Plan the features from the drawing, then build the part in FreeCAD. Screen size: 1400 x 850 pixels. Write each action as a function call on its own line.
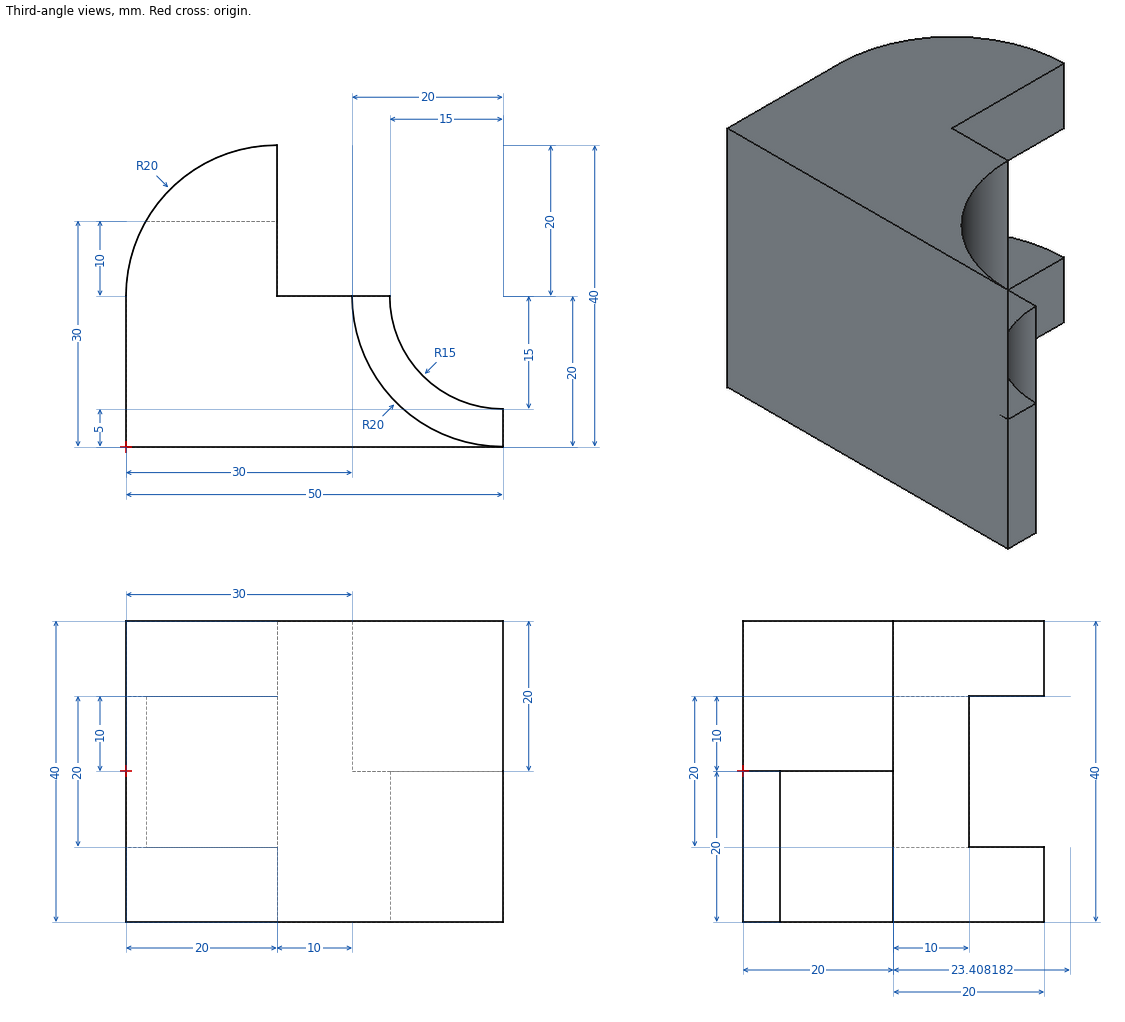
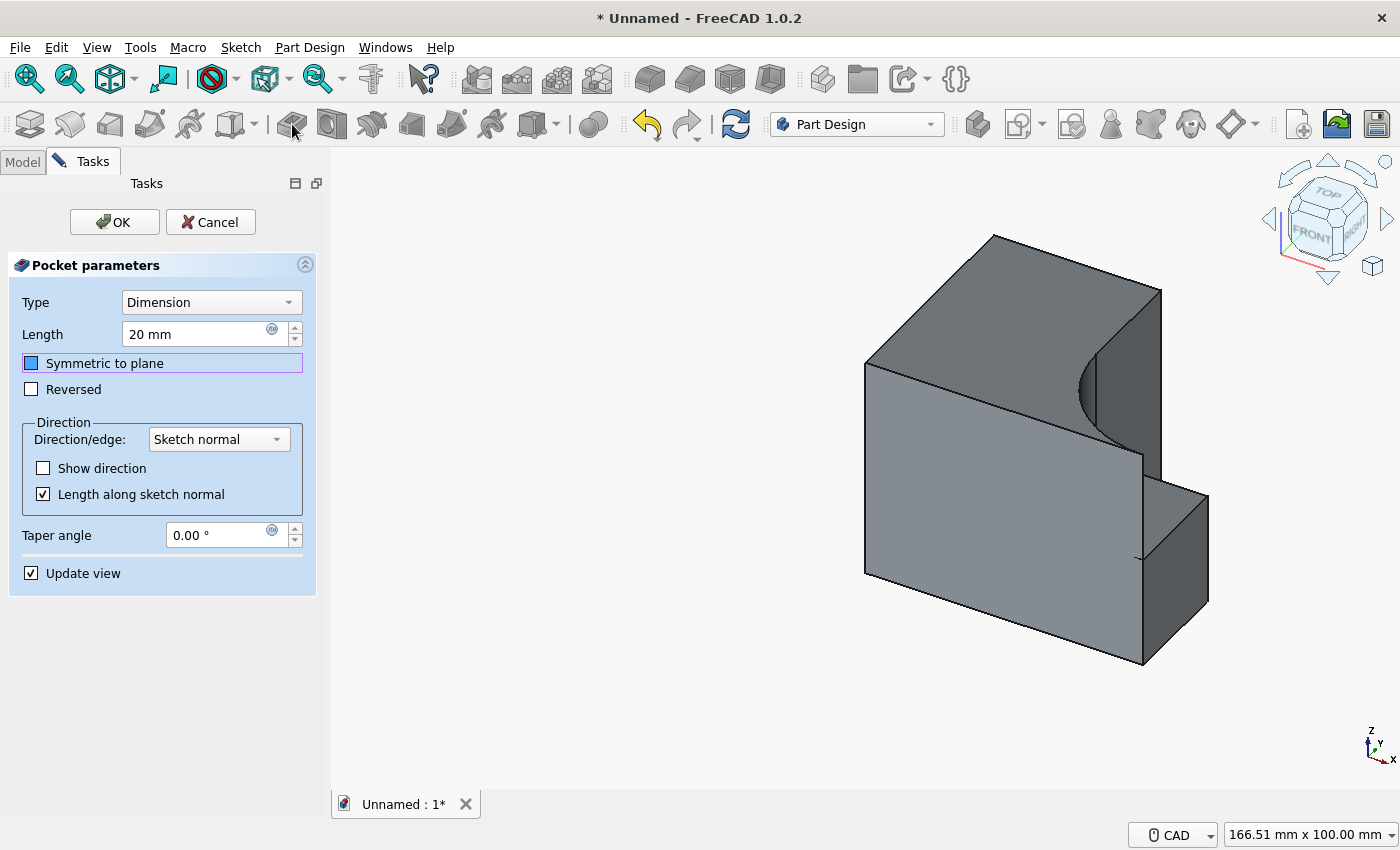
click(115, 222)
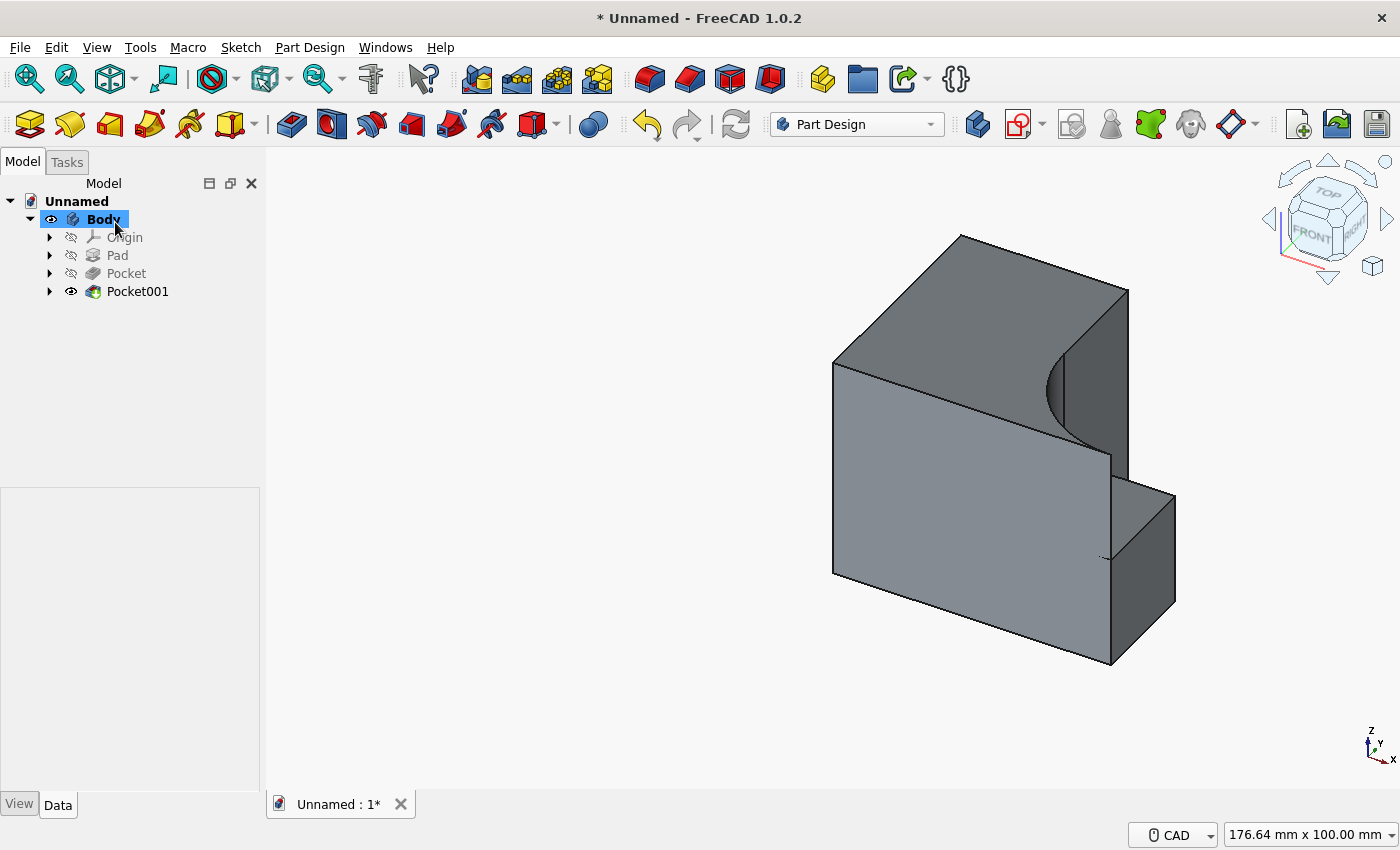
click(1122, 496)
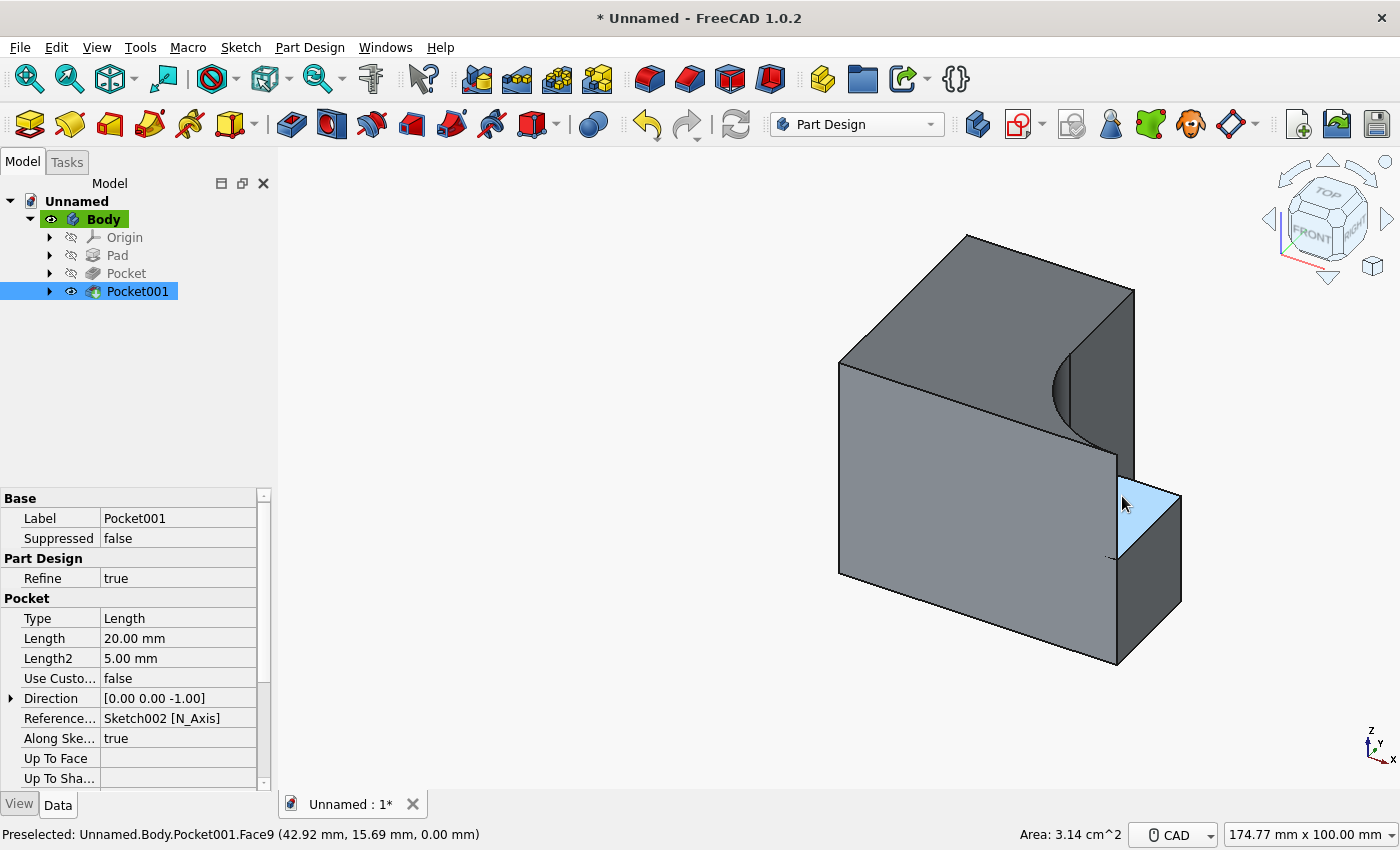
click(1018, 124)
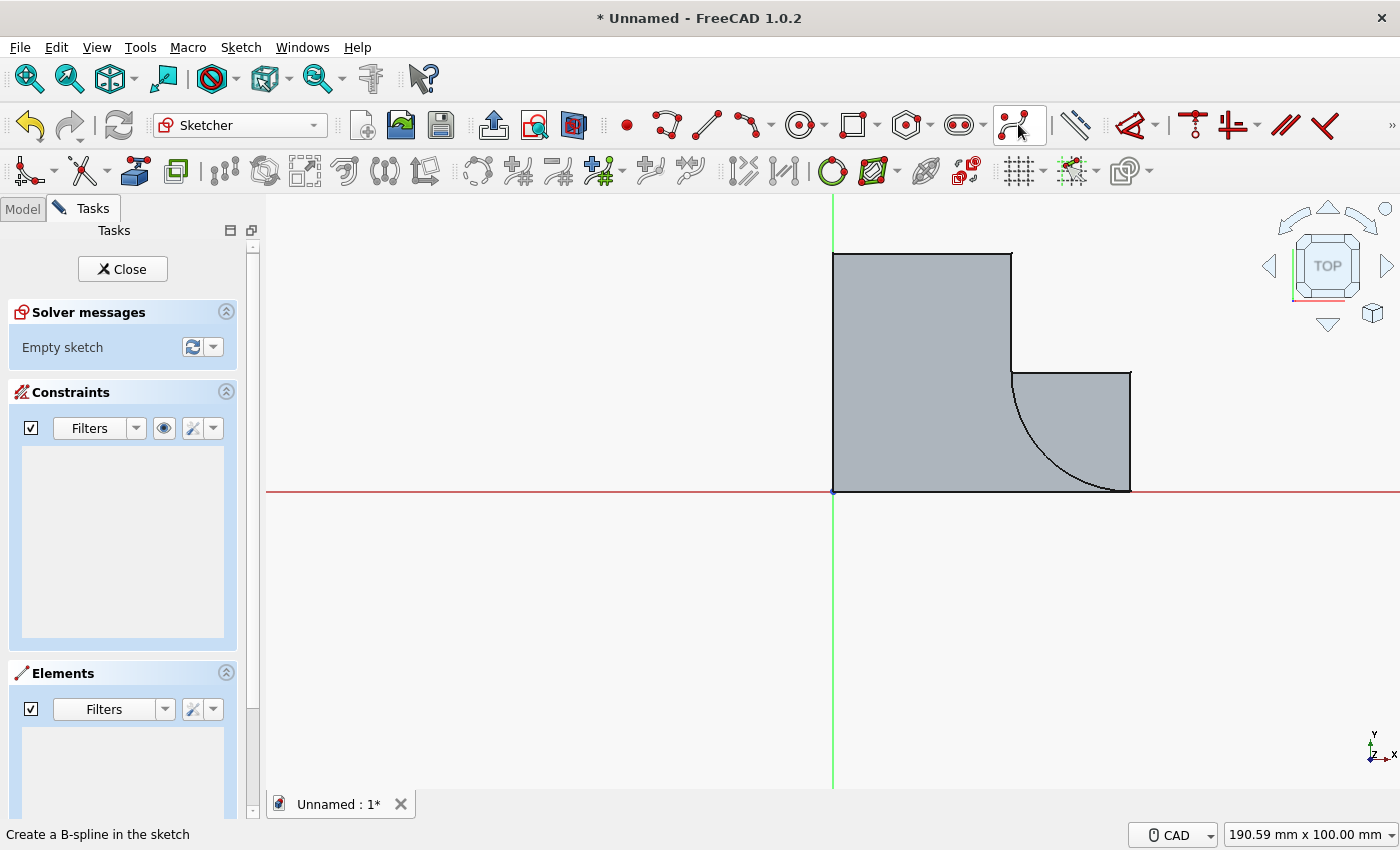
scroll(1191, 393, up, 7)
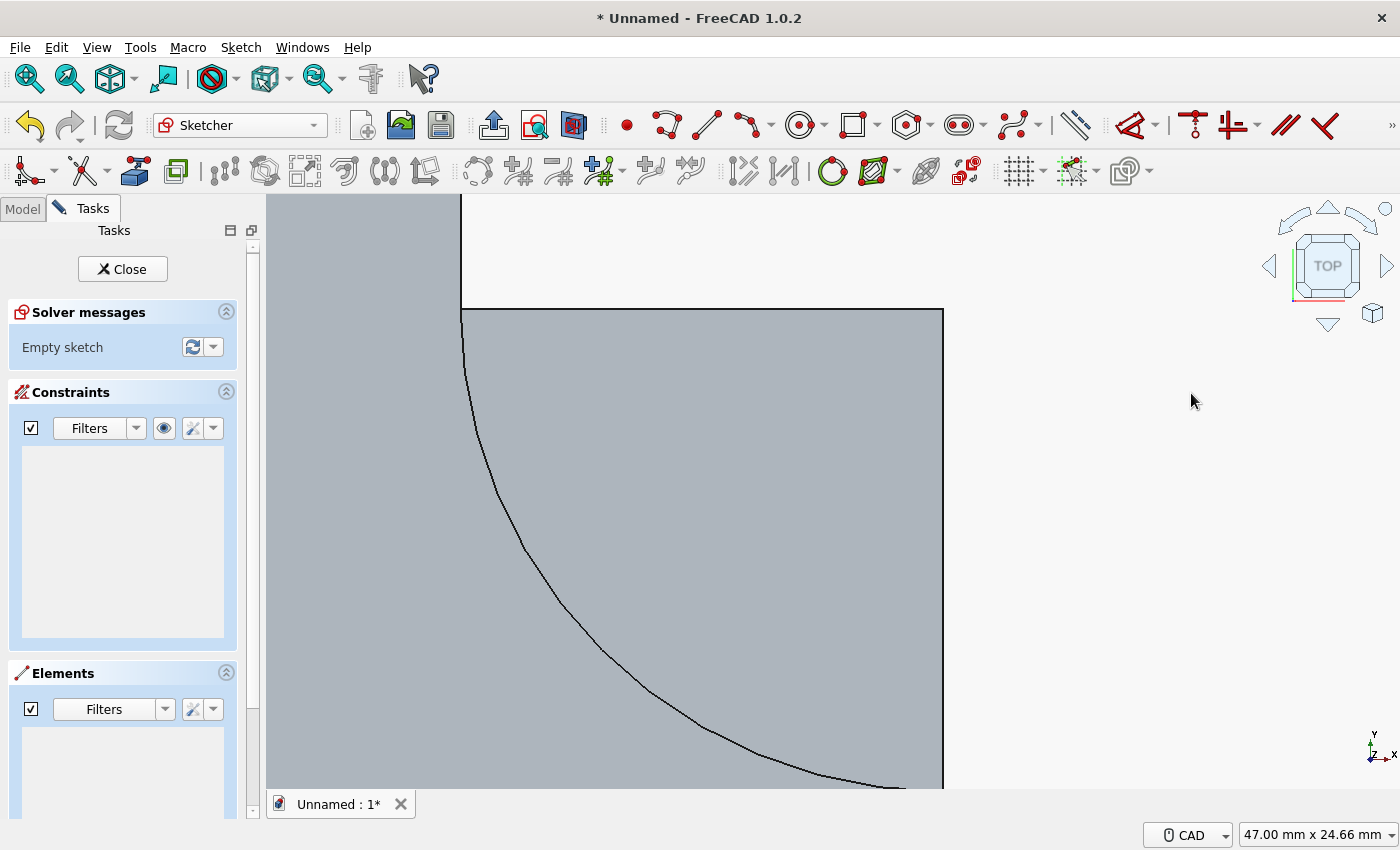
click(668, 126)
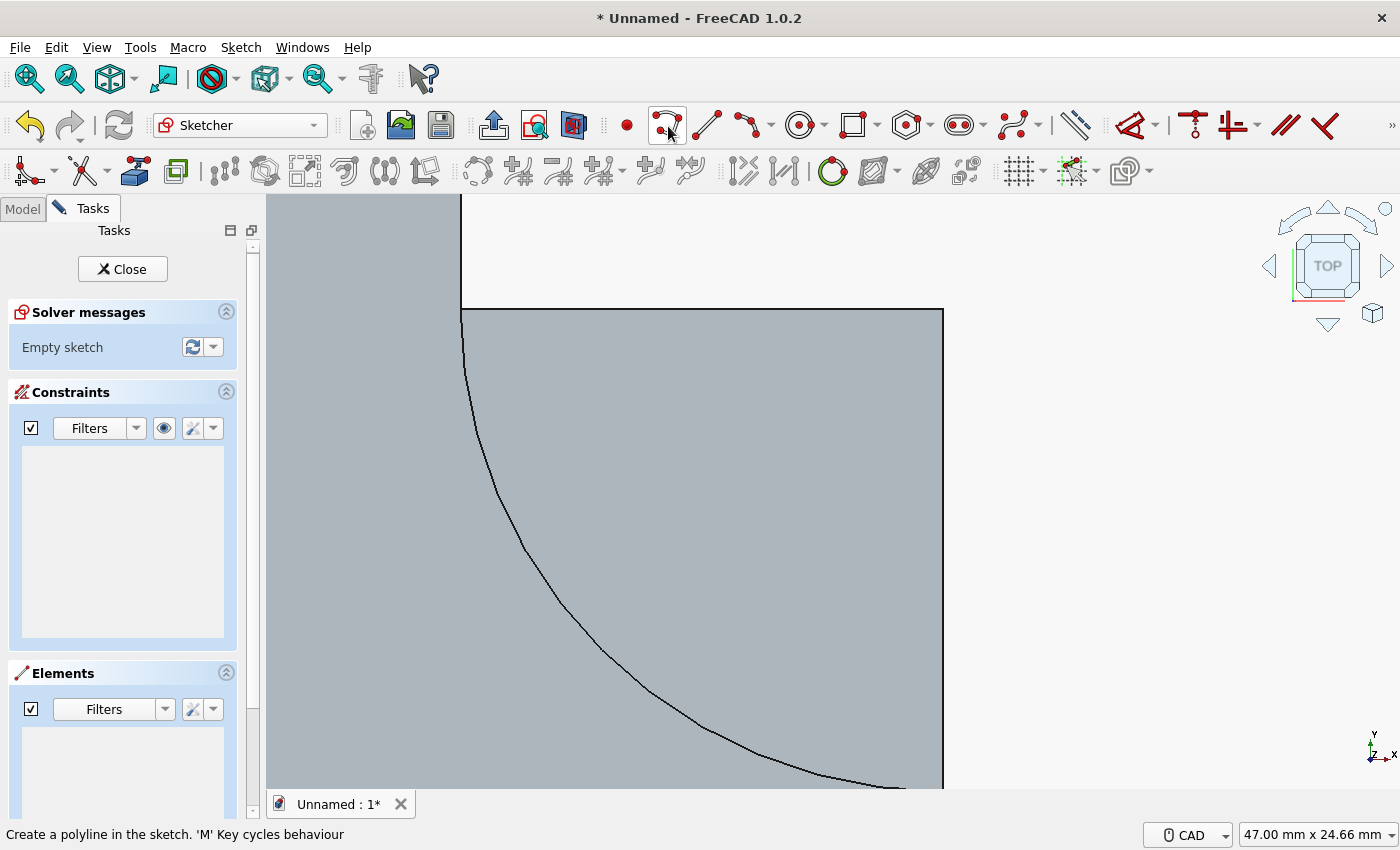
click(943, 671)
click(943, 309)
click(581, 309)
right_click(581, 309)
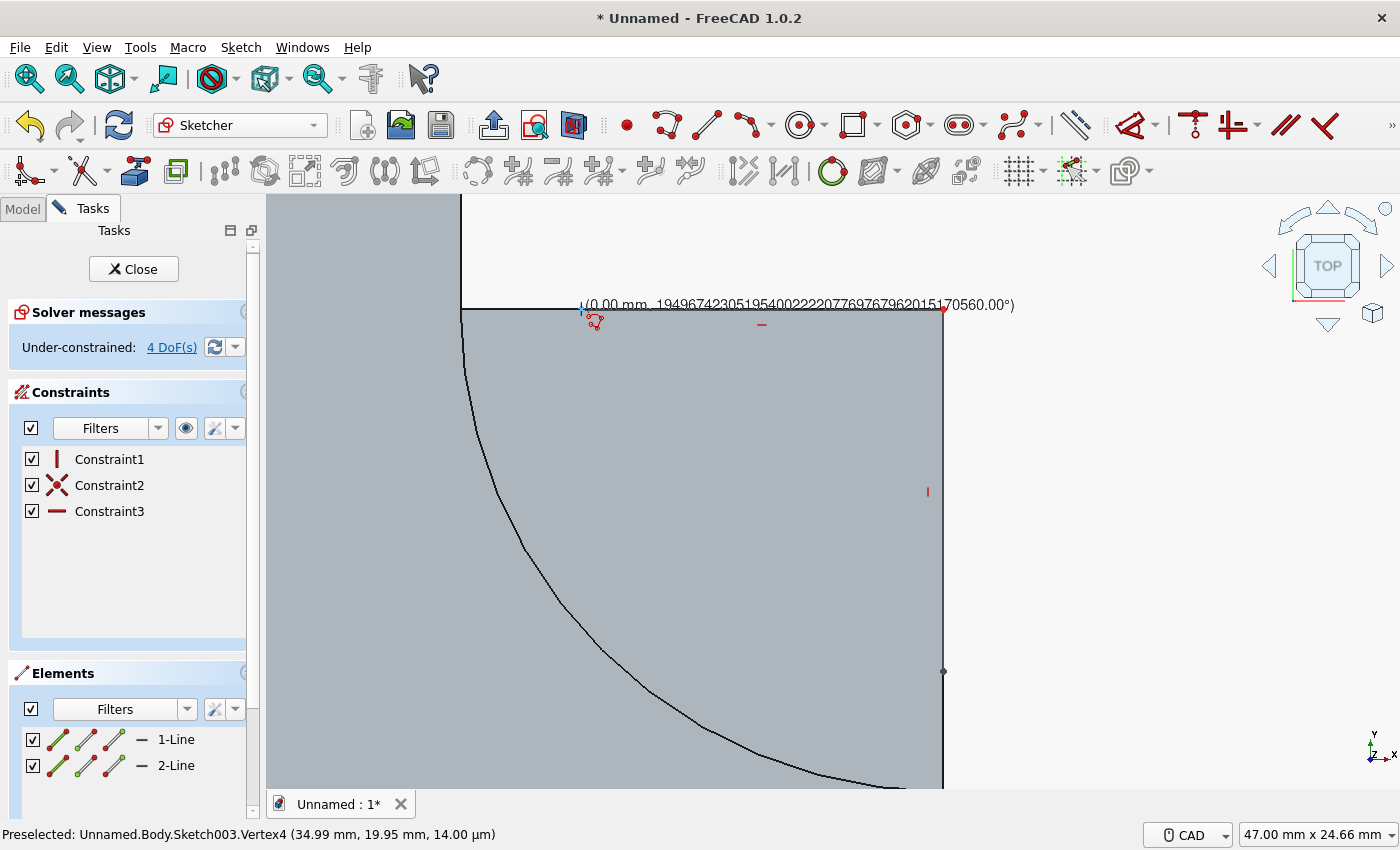
key(g)
key(3)
key(a)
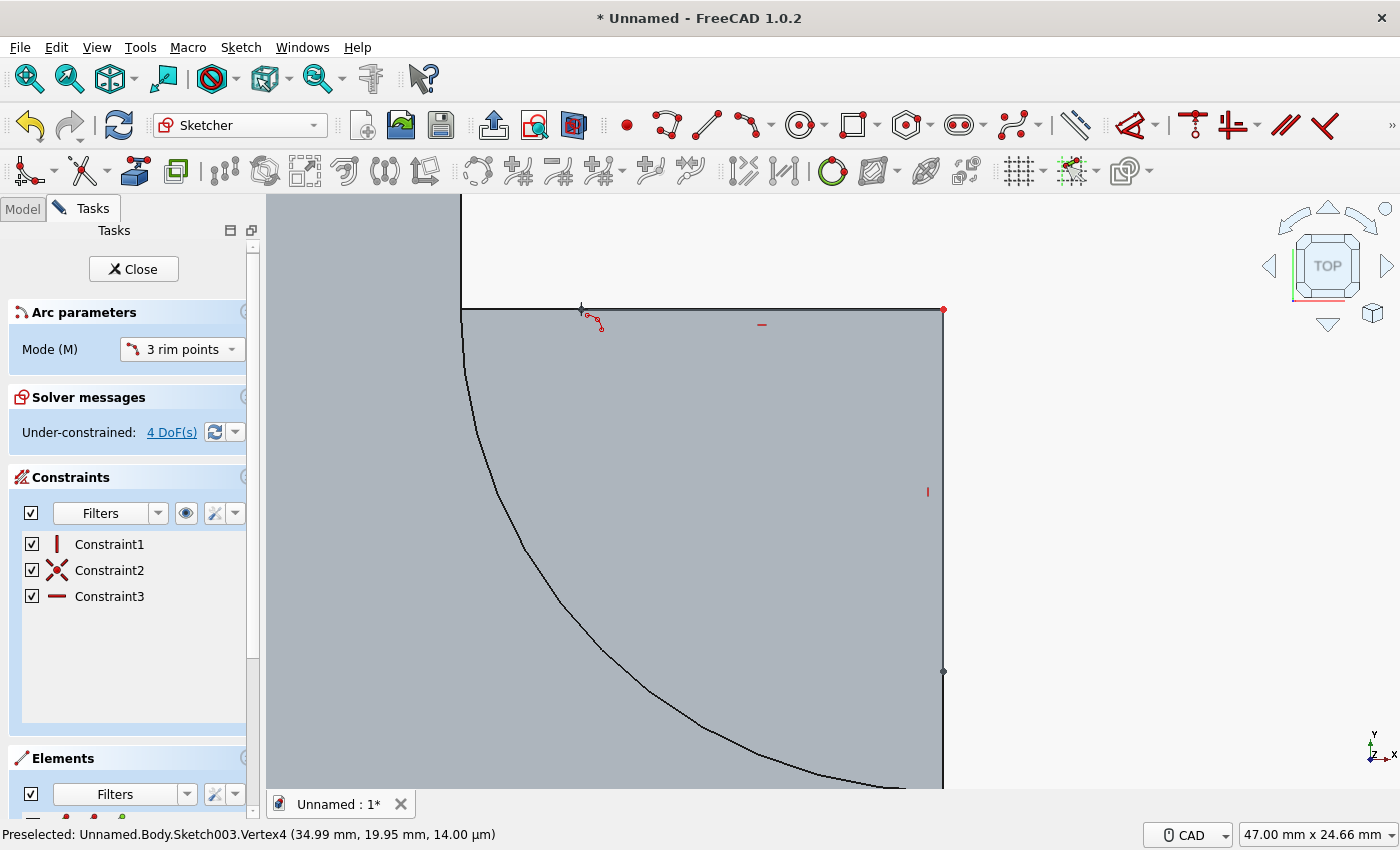
click(581, 310)
click(943, 672)
click(687, 565)
key(Escape)